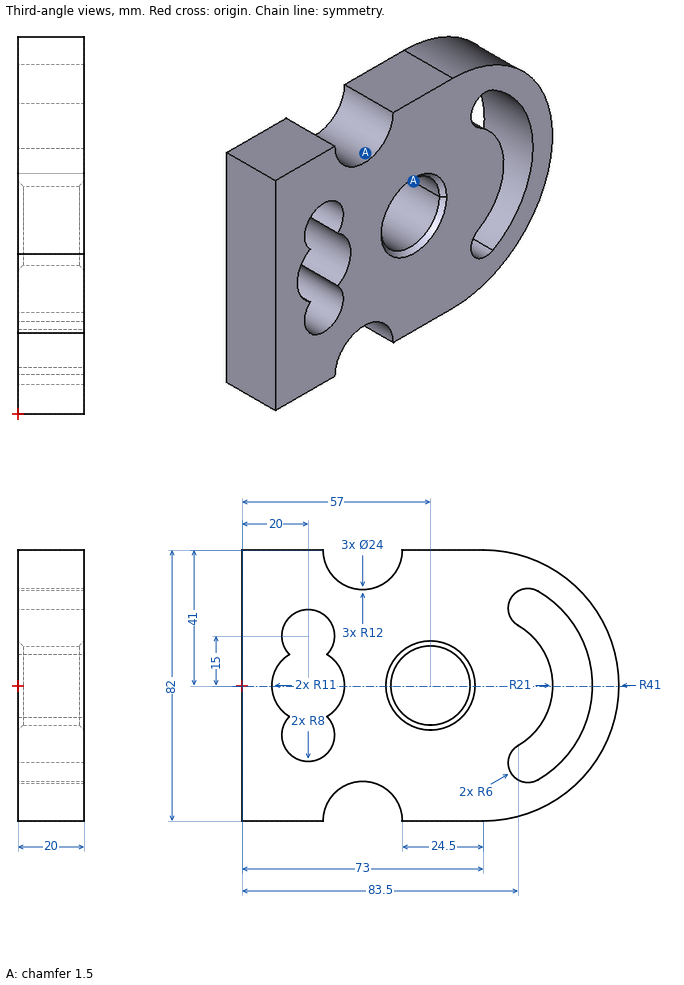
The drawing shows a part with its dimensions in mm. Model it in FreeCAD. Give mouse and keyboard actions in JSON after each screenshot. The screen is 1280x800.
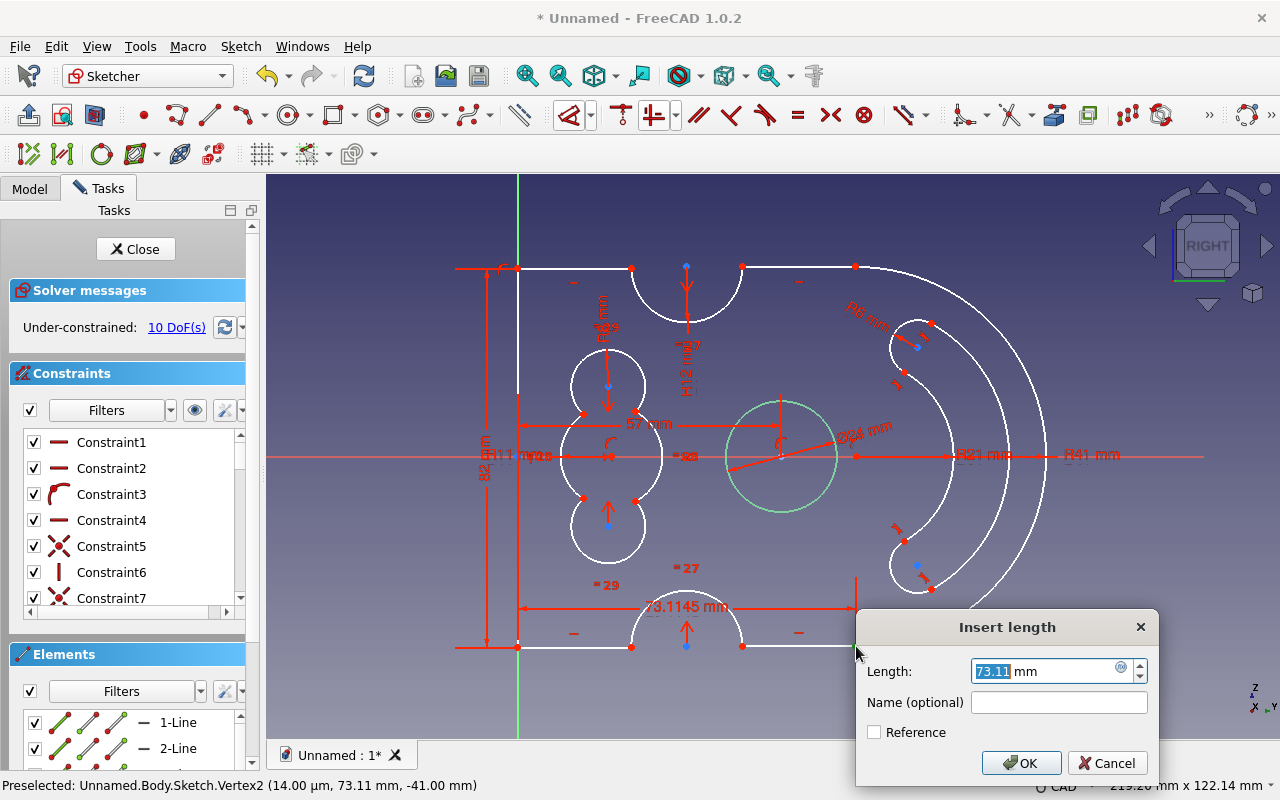
{"action": "type", "text": "73"}
{"action": "key", "text": "Return"}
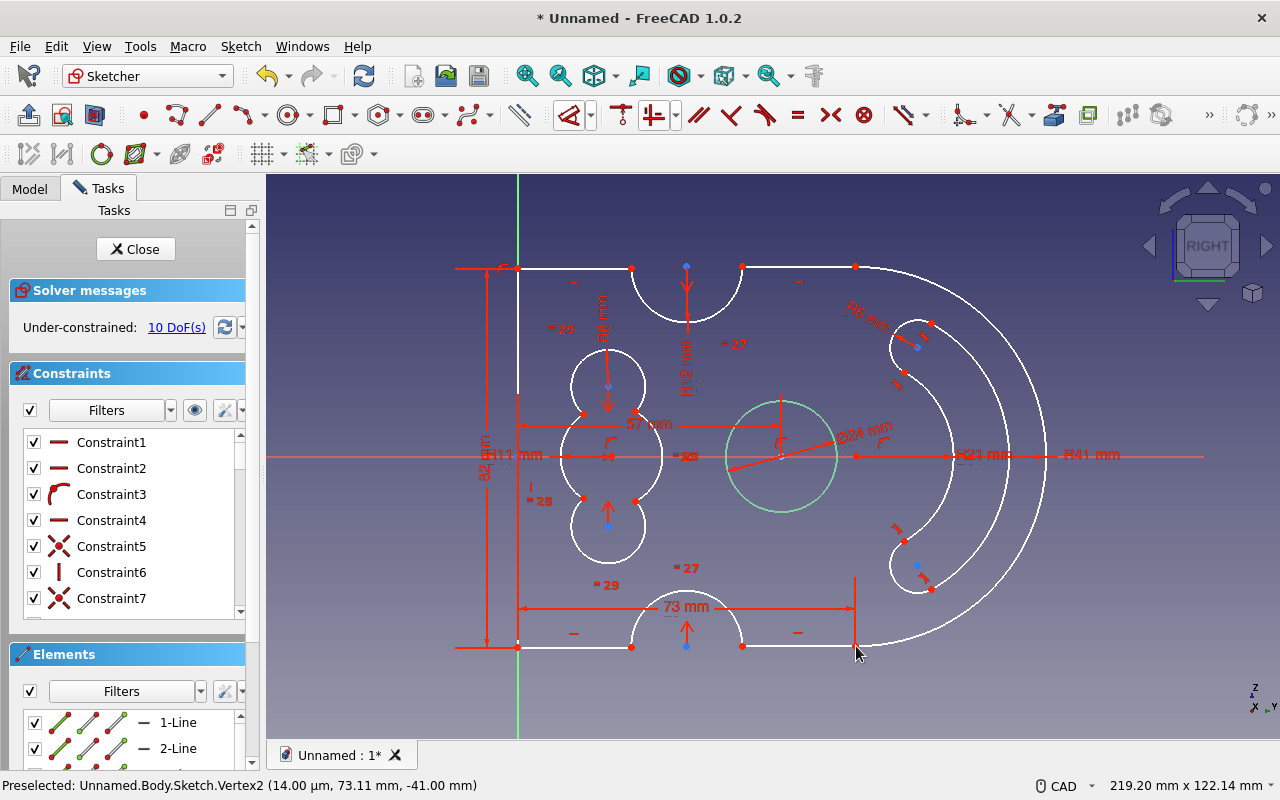
{"action": "left_click", "coordinate": [856, 267]}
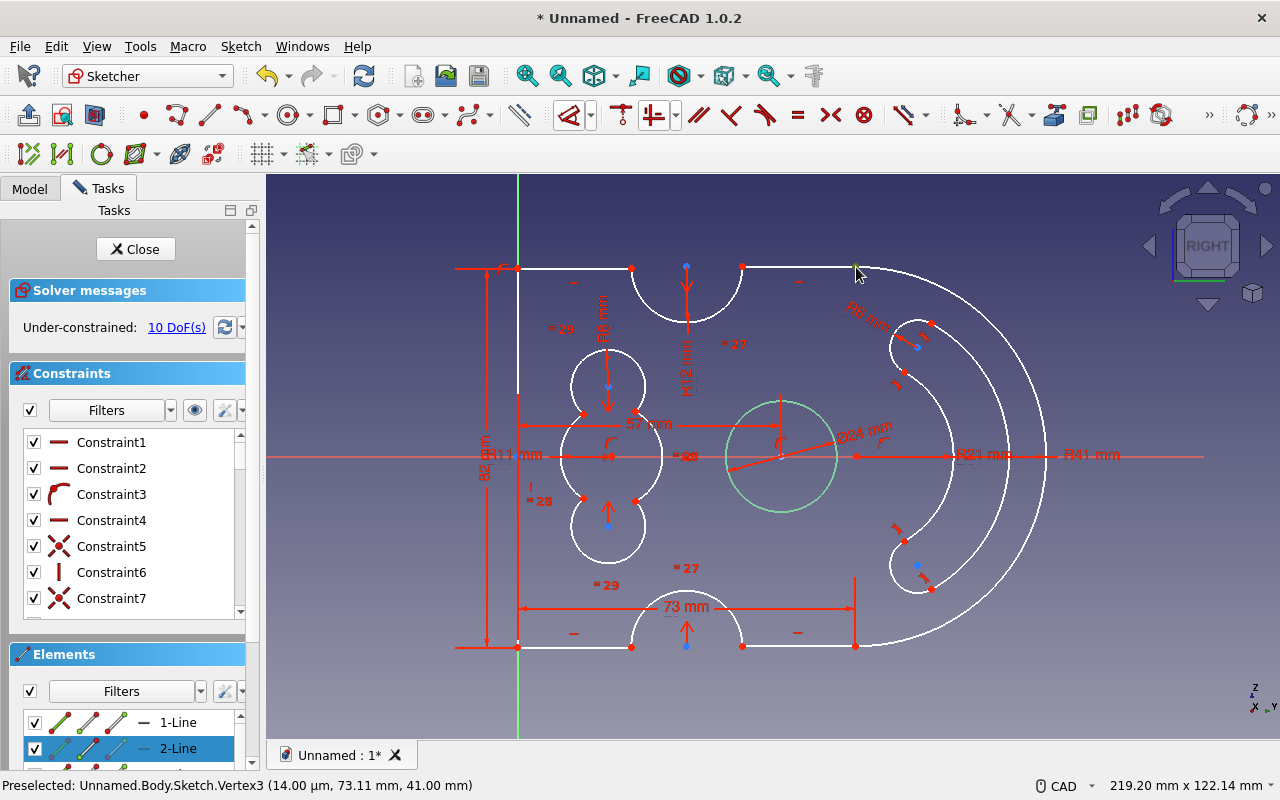
{"action": "key", "text": "l"}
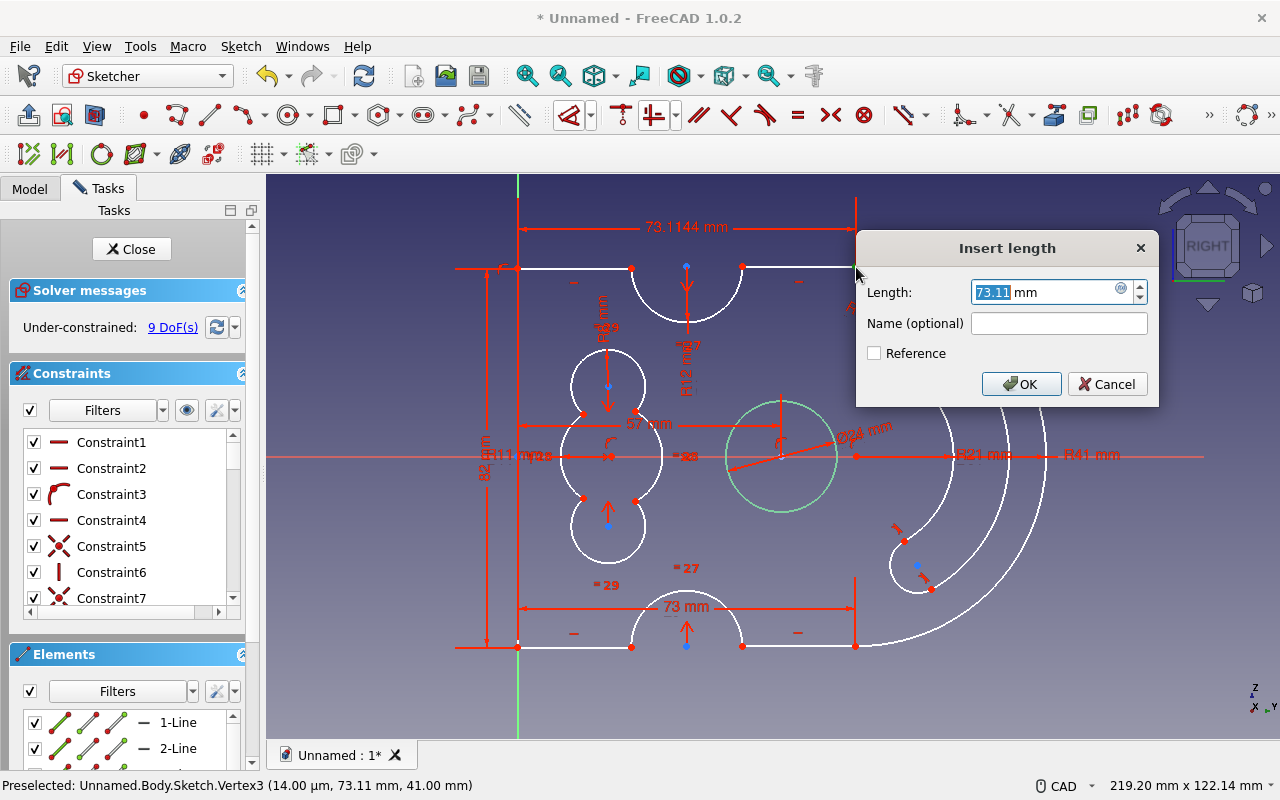
{"action": "type", "text": "73"}
{"action": "key", "text": "Return"}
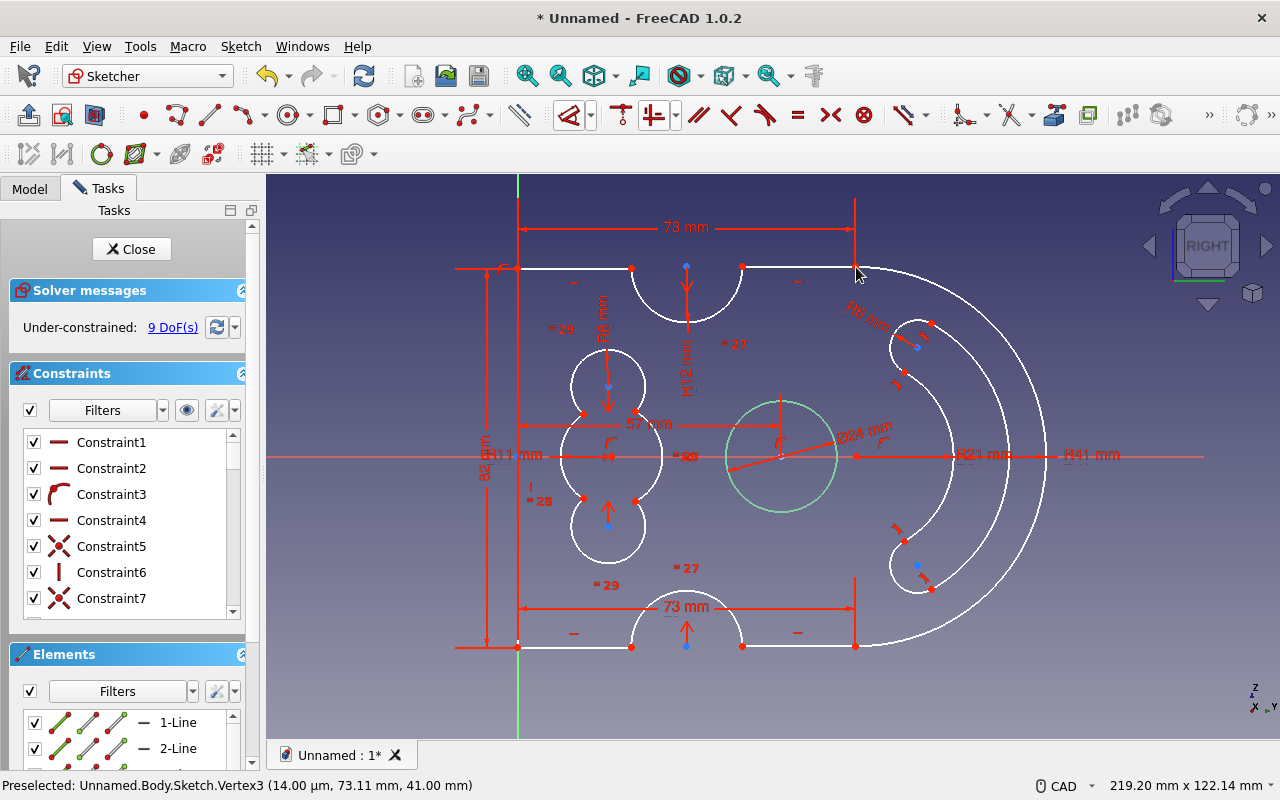
{"action": "left_click", "coordinate": [631, 269]}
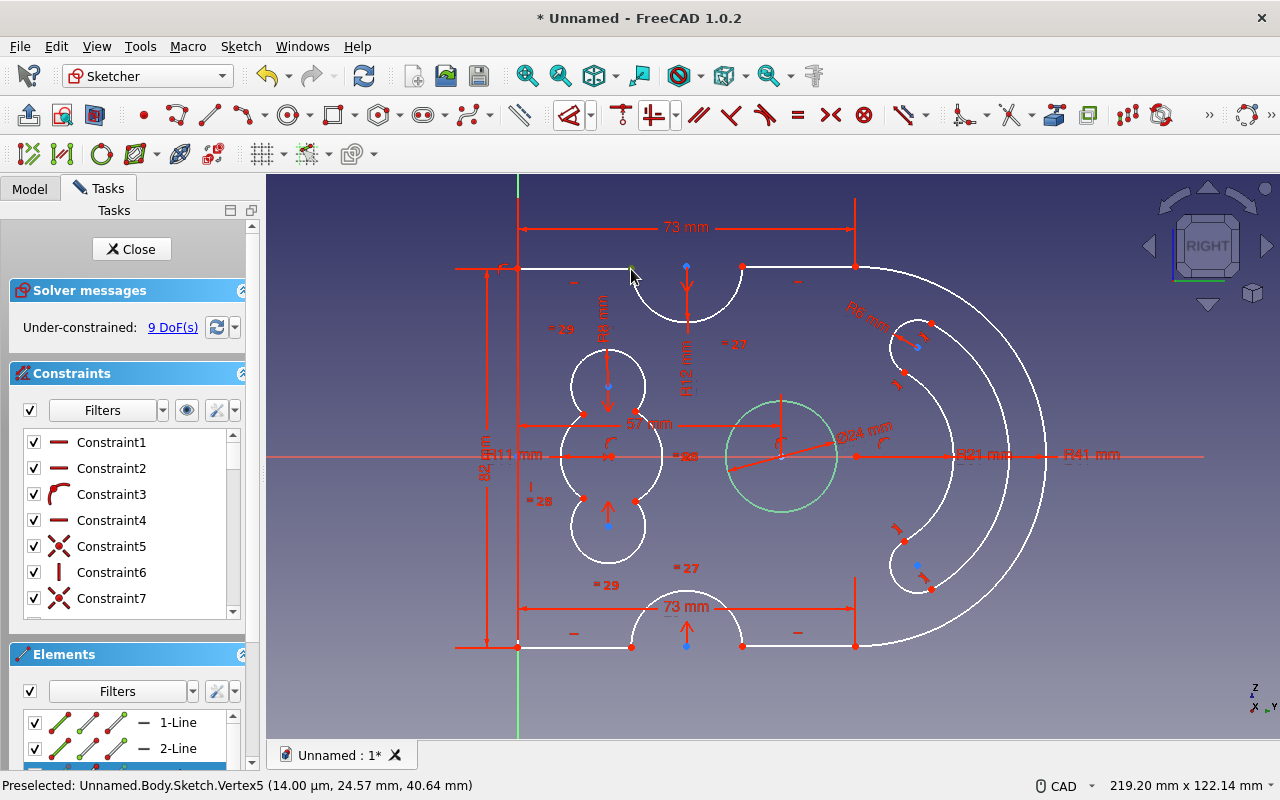
{"action": "left_click", "coordinate": [590, 116]}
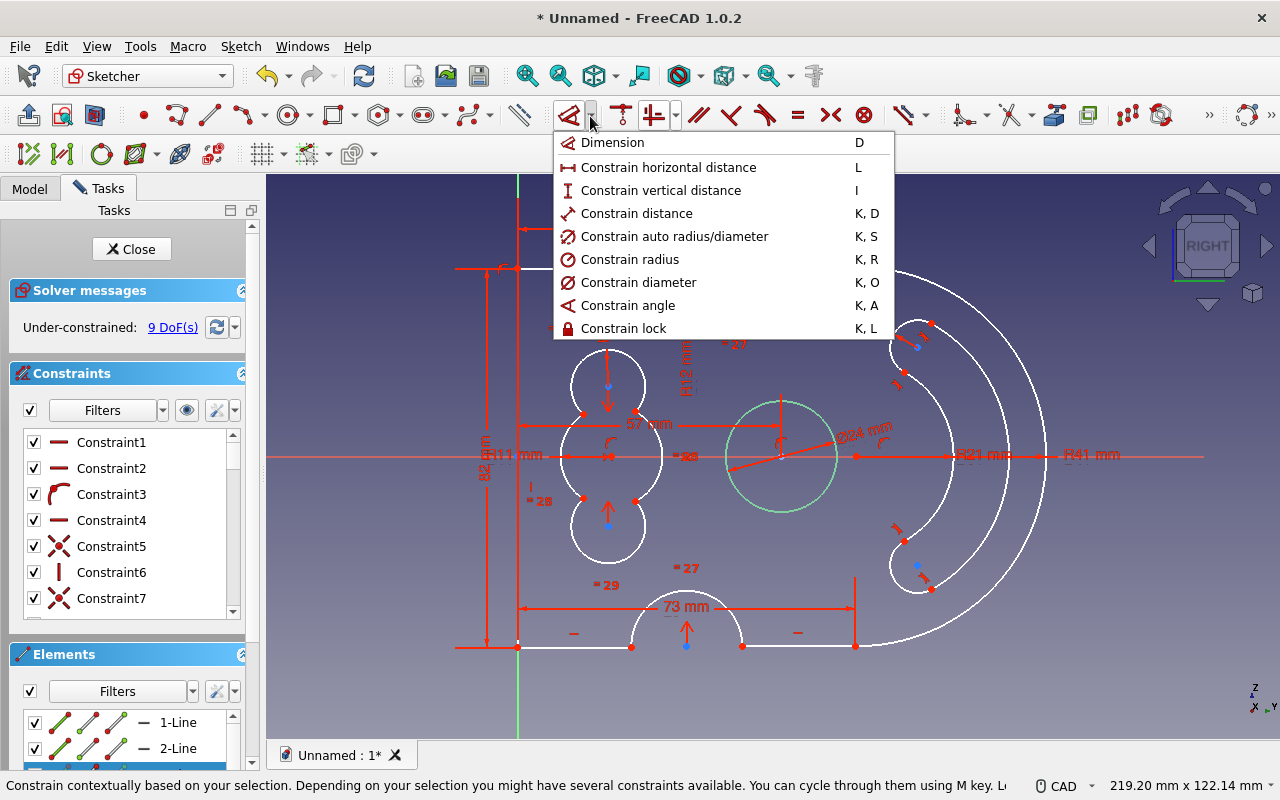
{"action": "left_click", "coordinate": [724, 190]}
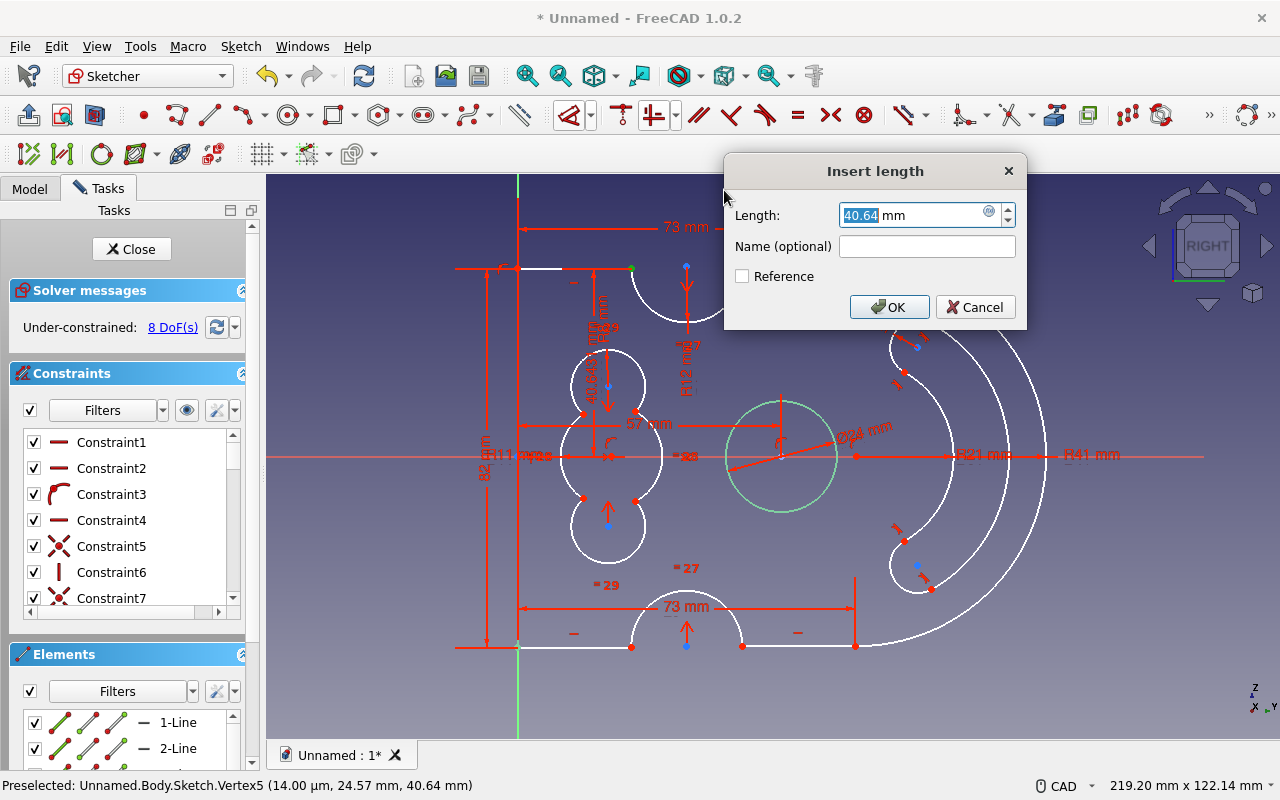
{"action": "type", "text": "41"}
{"action": "key", "text": "Return"}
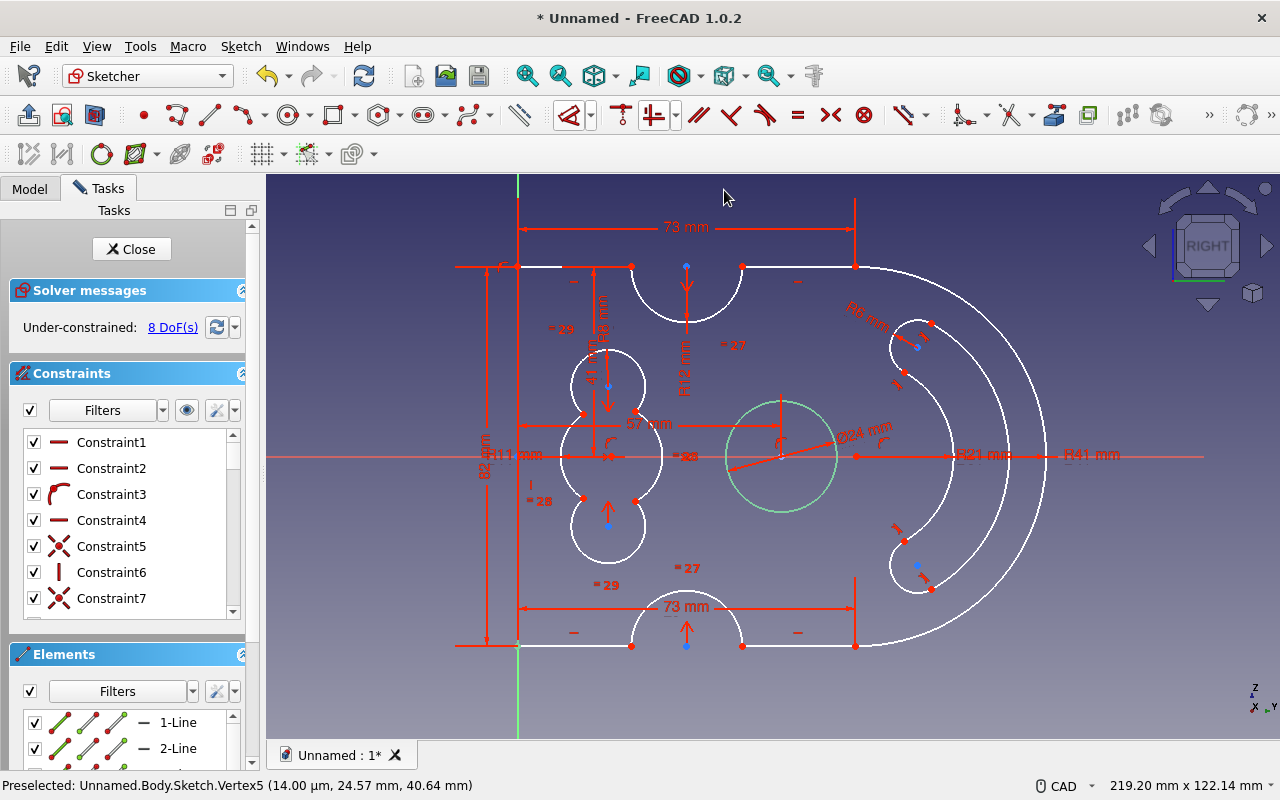
{"action": "left_click", "coordinate": [856, 457]}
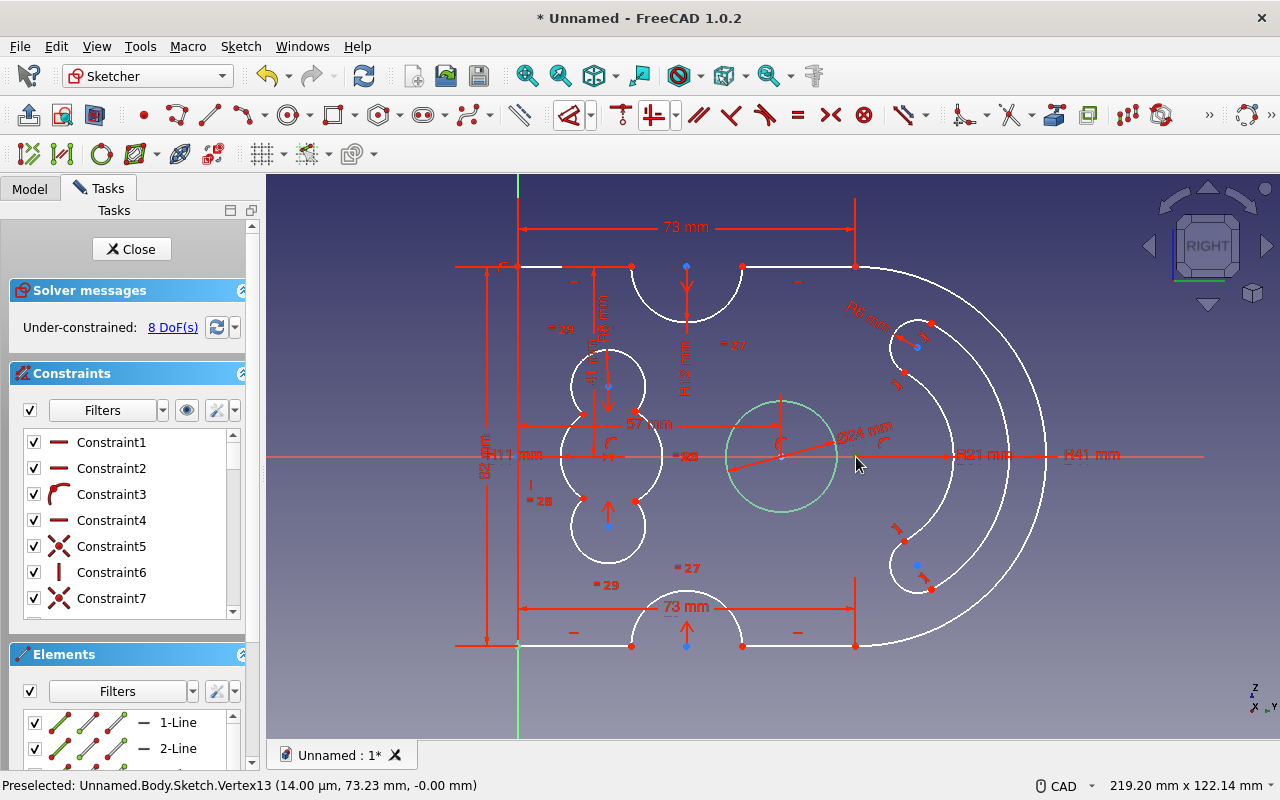
{"action": "key", "text": "l"}